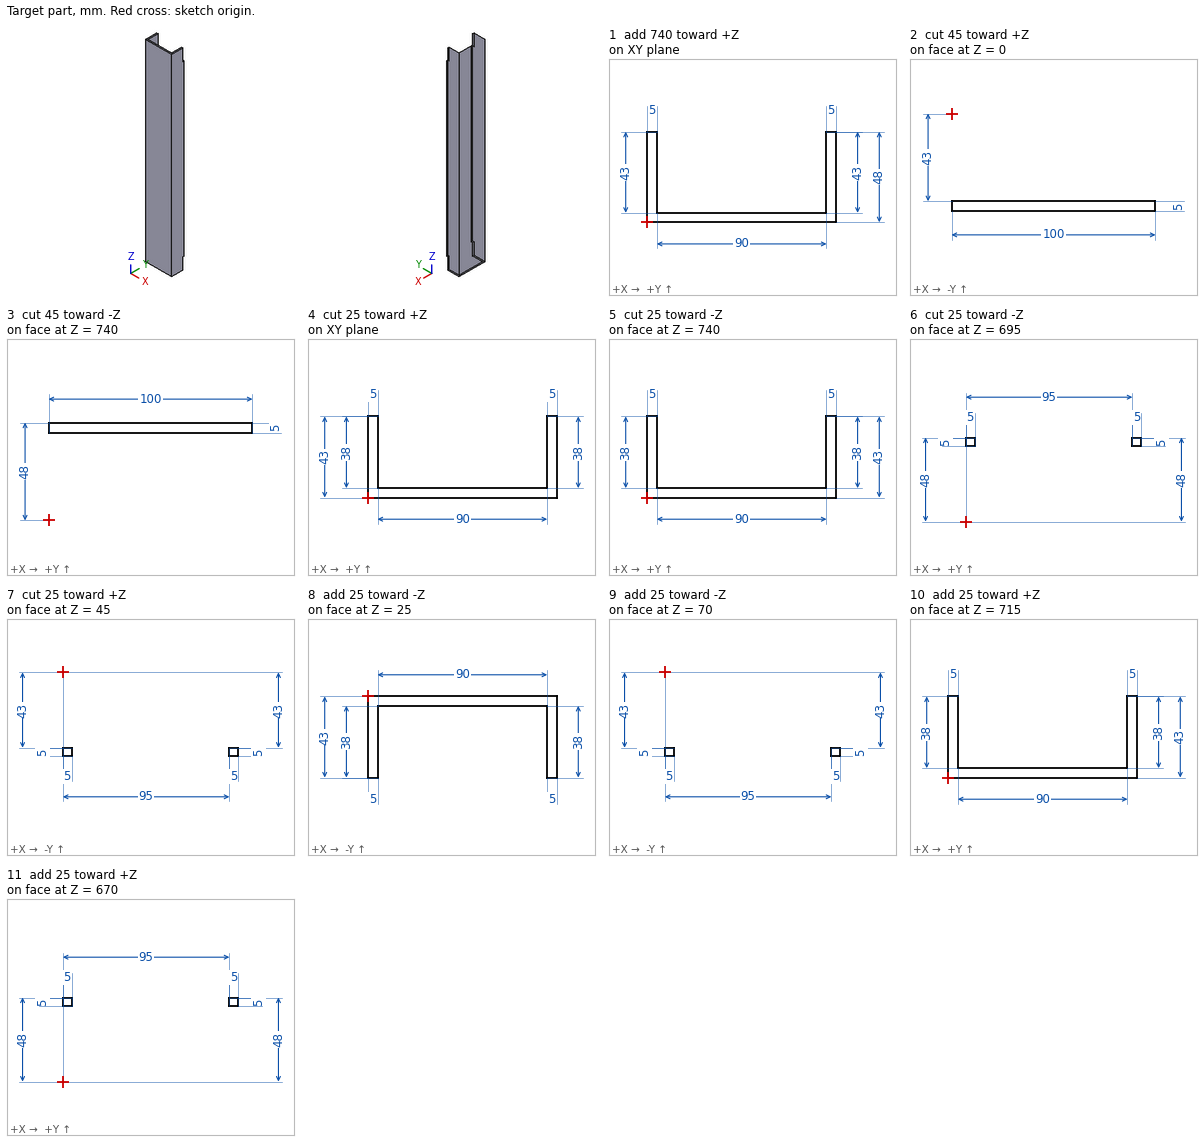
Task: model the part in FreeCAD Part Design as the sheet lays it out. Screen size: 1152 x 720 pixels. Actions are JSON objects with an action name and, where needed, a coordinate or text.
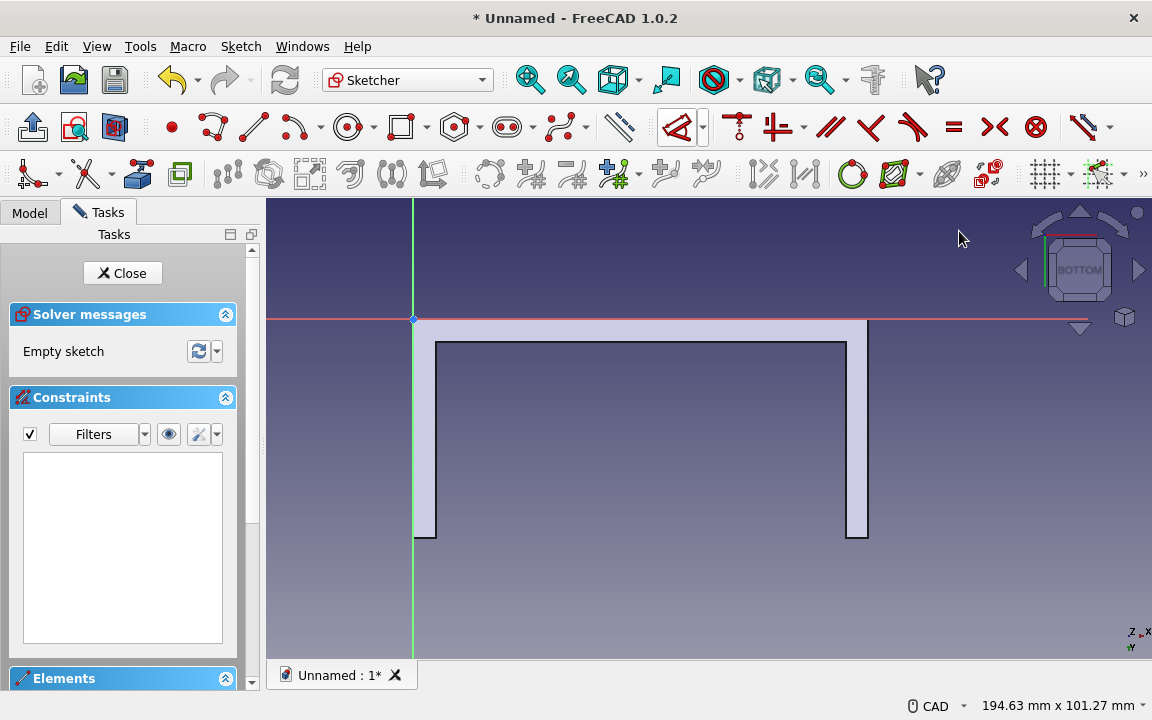
{"action": "left_click", "coordinate": [400, 128]}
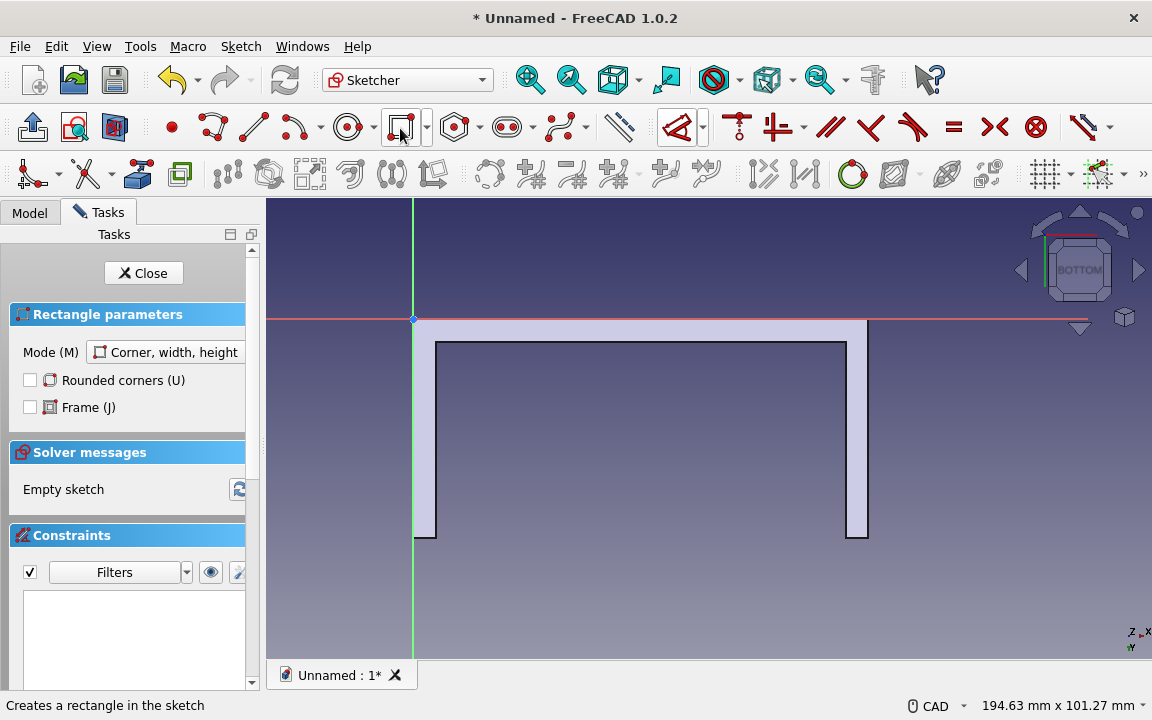
{"action": "left_click", "coordinate": [413, 515]}
{"action": "mouse_move", "coordinate": [868, 538]}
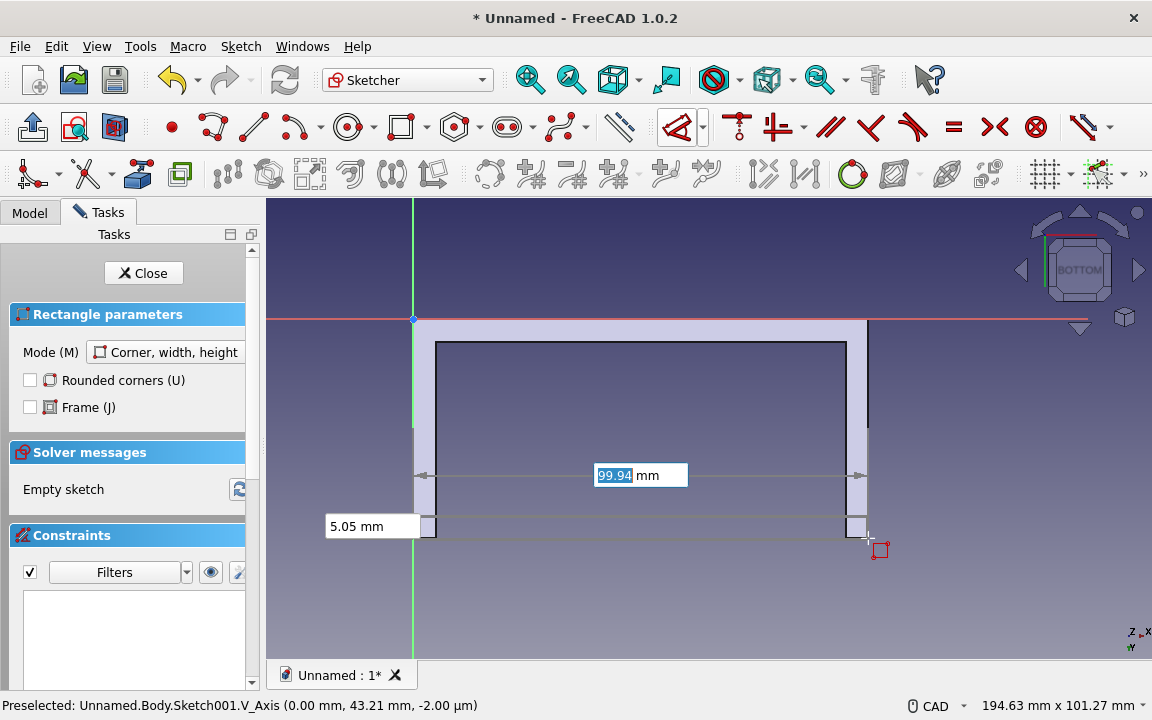
{"action": "type", "text": "100"}
{"action": "key", "text": "Tab"}
{"action": "type", "text": "5"}
{"action": "key", "text": "Return"}
{"action": "key", "text": "Escape"}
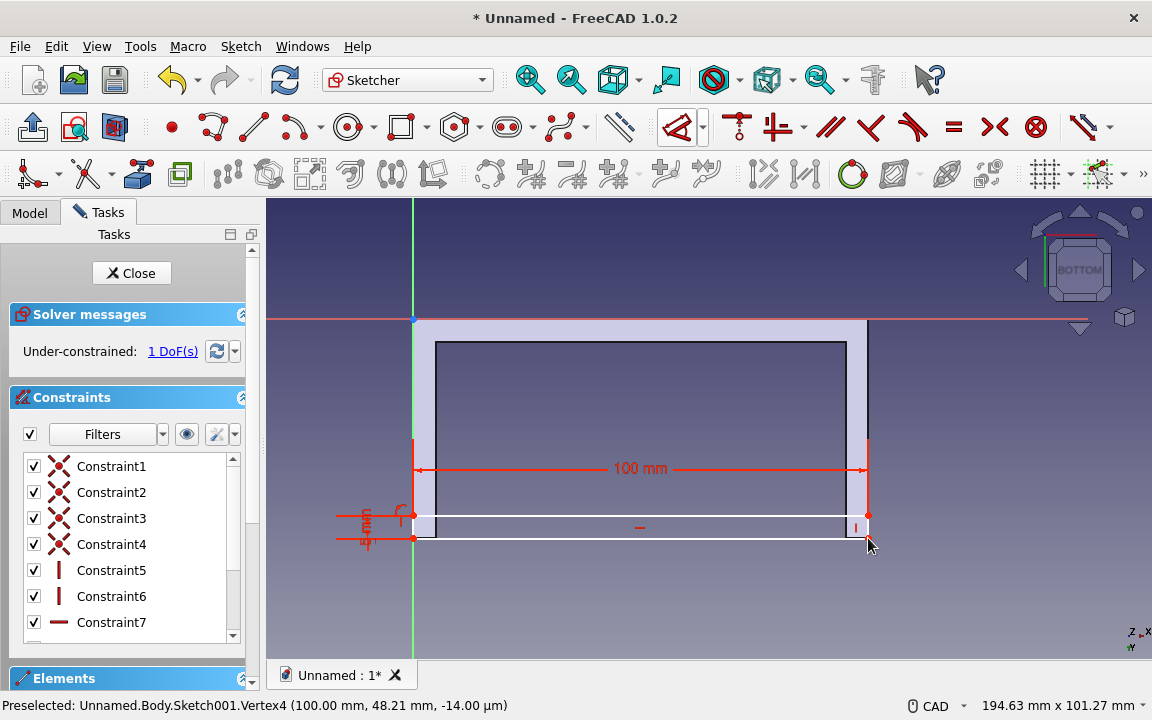
{"action": "left_click", "coordinate": [413, 516]}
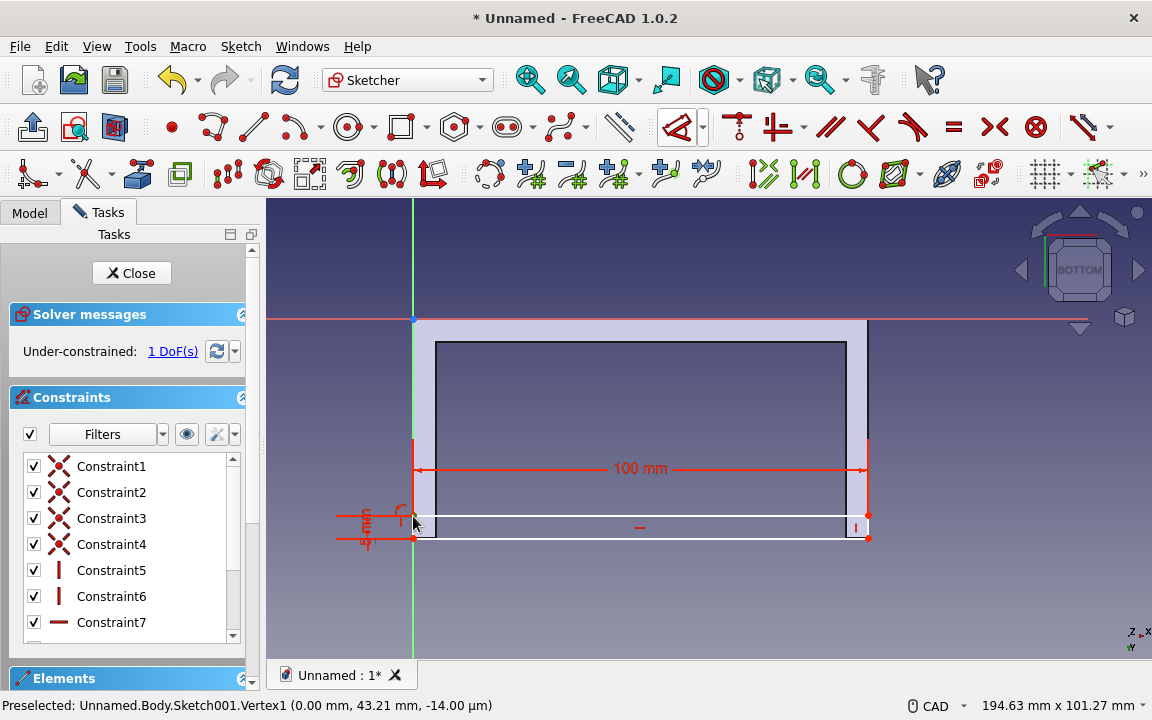
{"action": "left_click", "coordinate": [702, 128]}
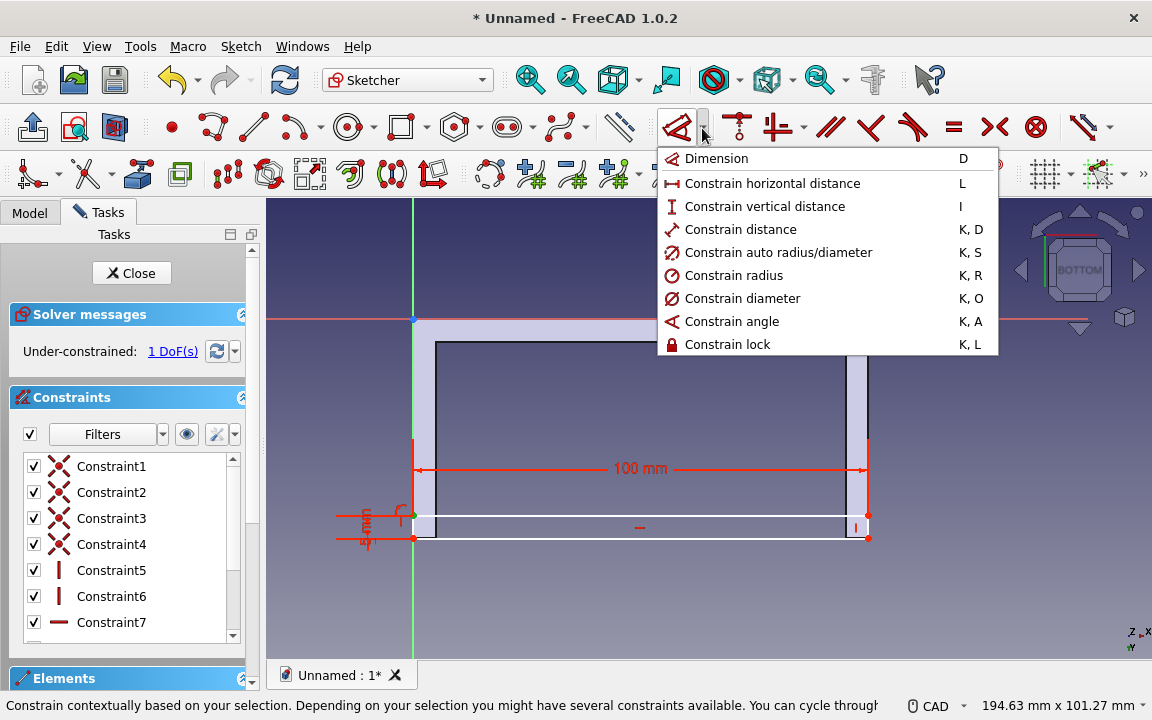
{"action": "left_click", "coordinate": [828, 206]}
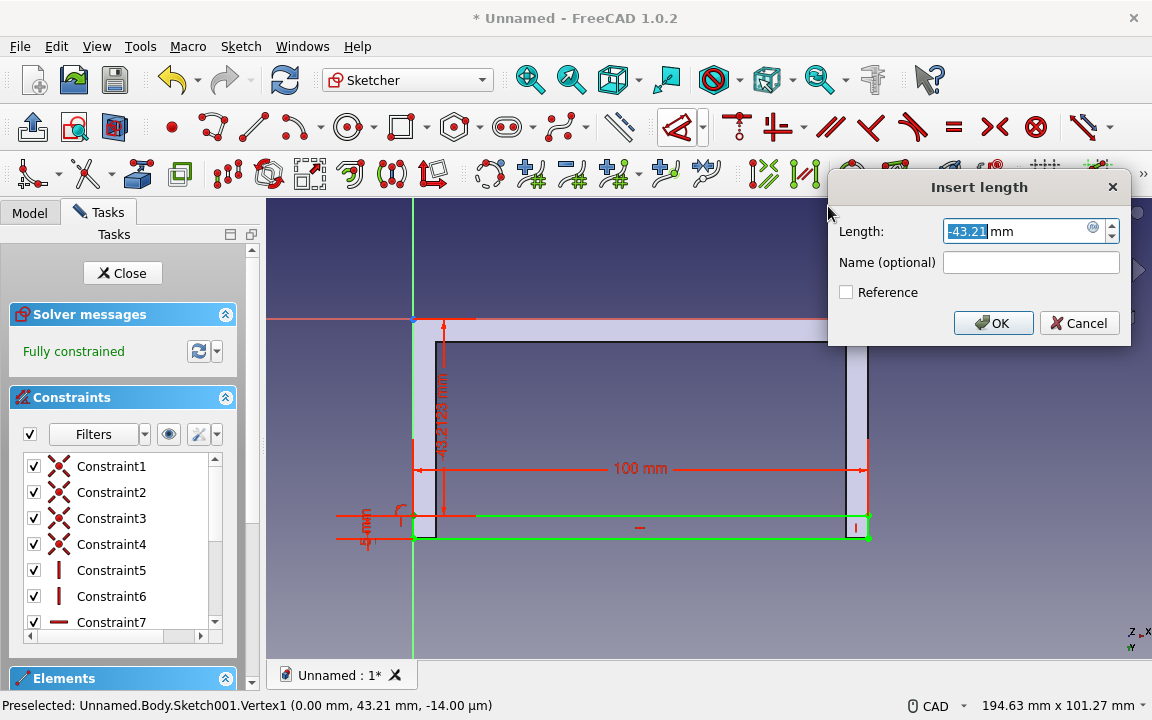
{"action": "type", "text": "-43"}
{"action": "key", "text": "Return"}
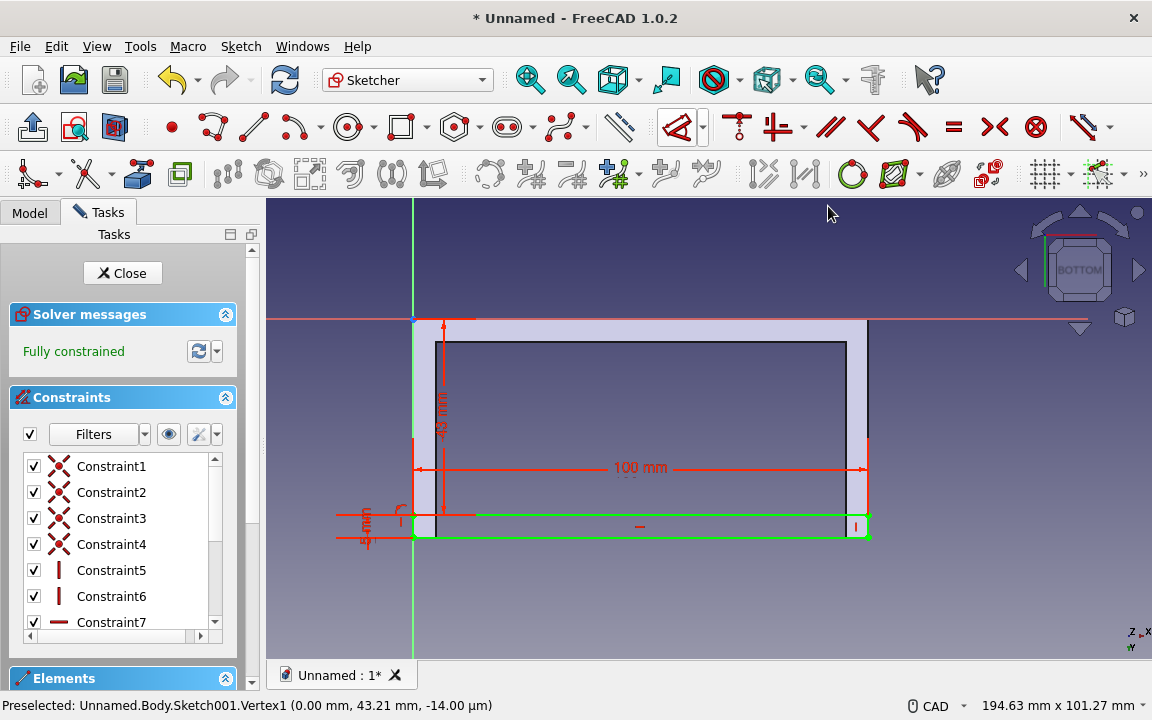
{"action": "left_click", "coordinate": [123, 273]}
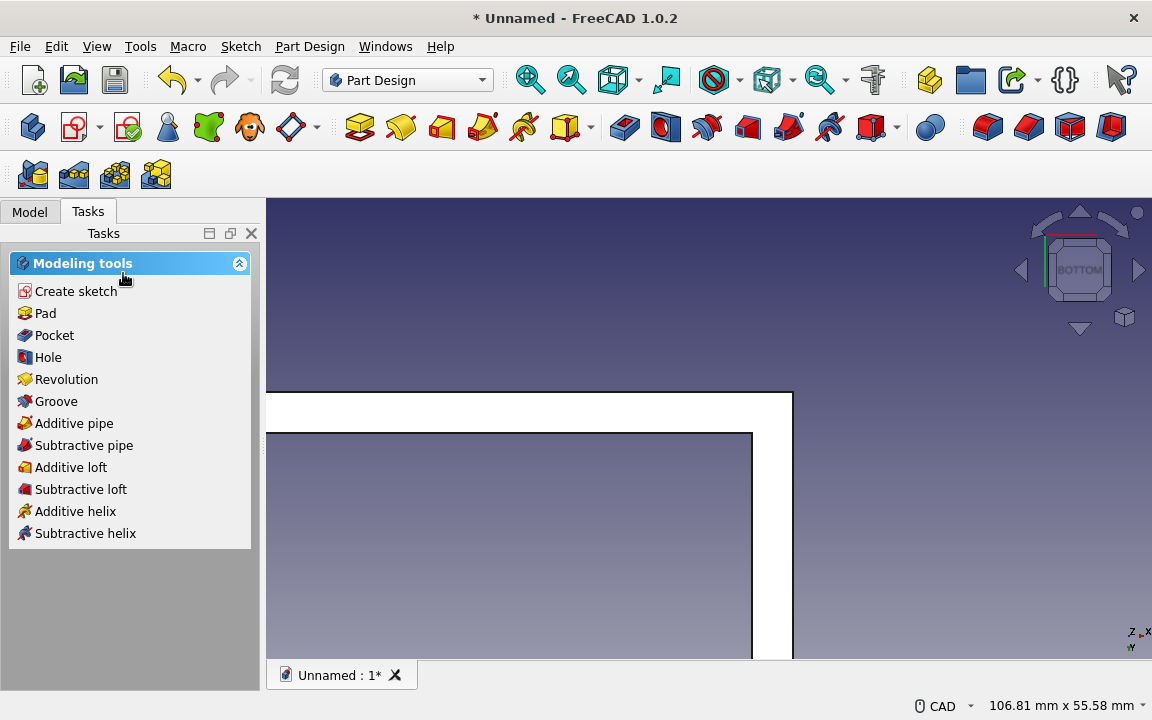
{"action": "left_click", "coordinate": [625, 128]}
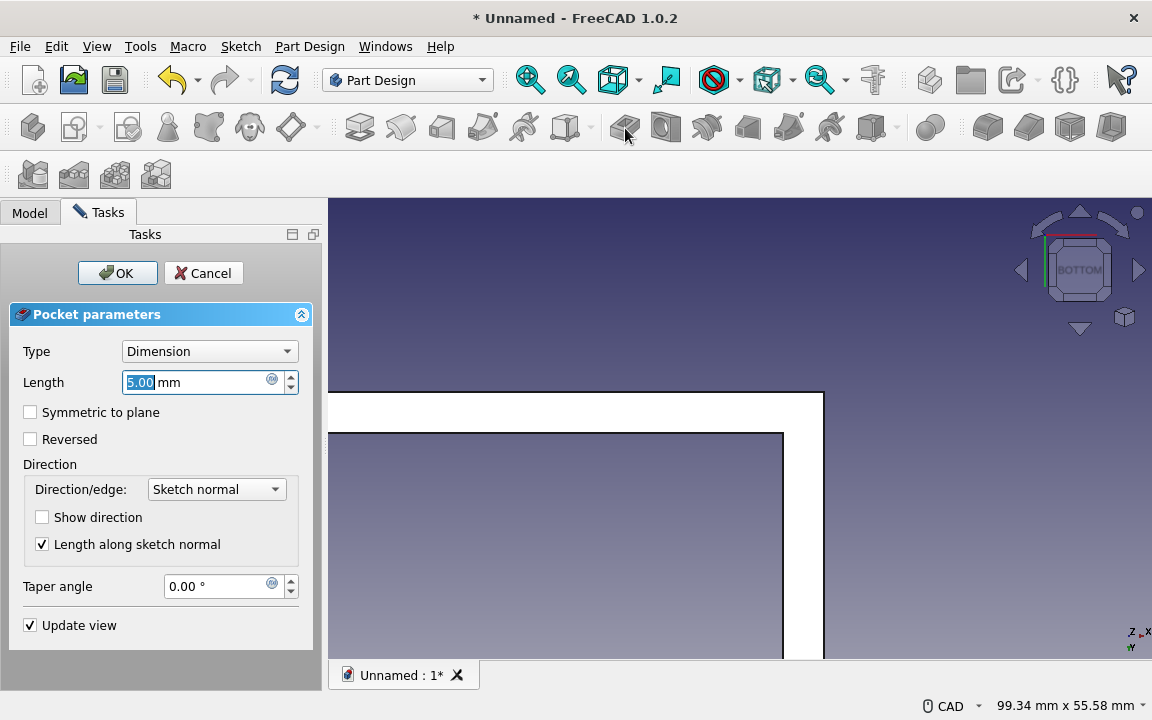
{"action": "type", "text": "45"}
{"action": "key", "text": "Tab"}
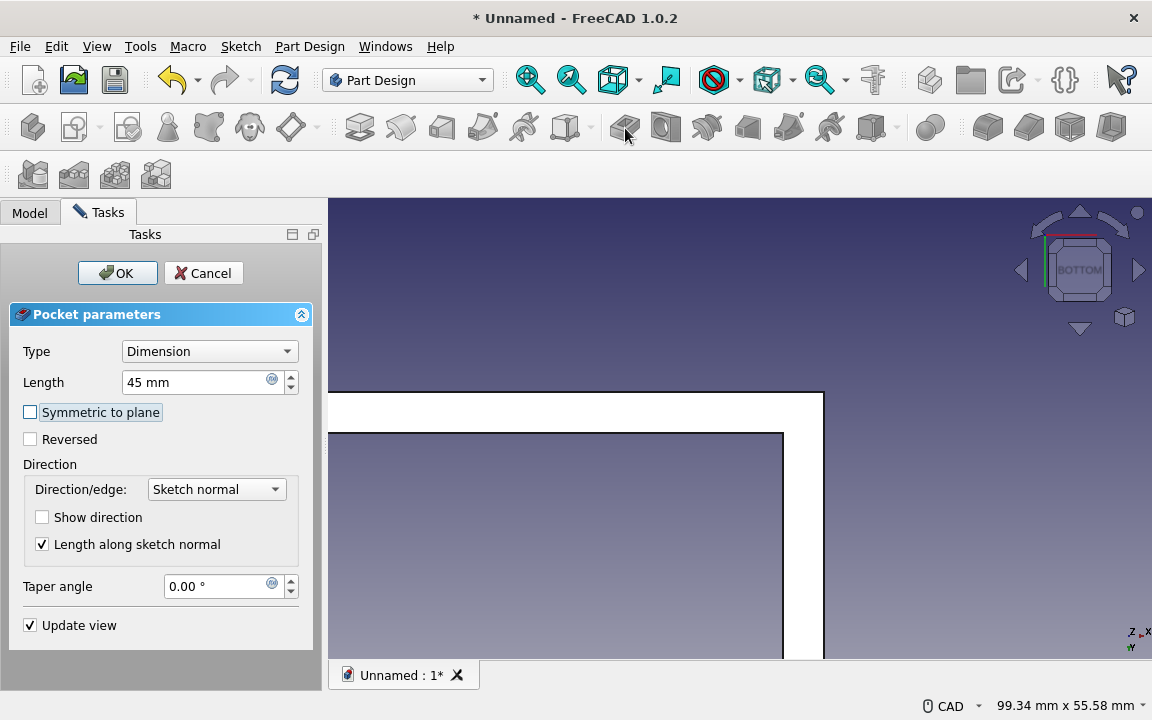
{"action": "left_click", "coordinate": [118, 273]}